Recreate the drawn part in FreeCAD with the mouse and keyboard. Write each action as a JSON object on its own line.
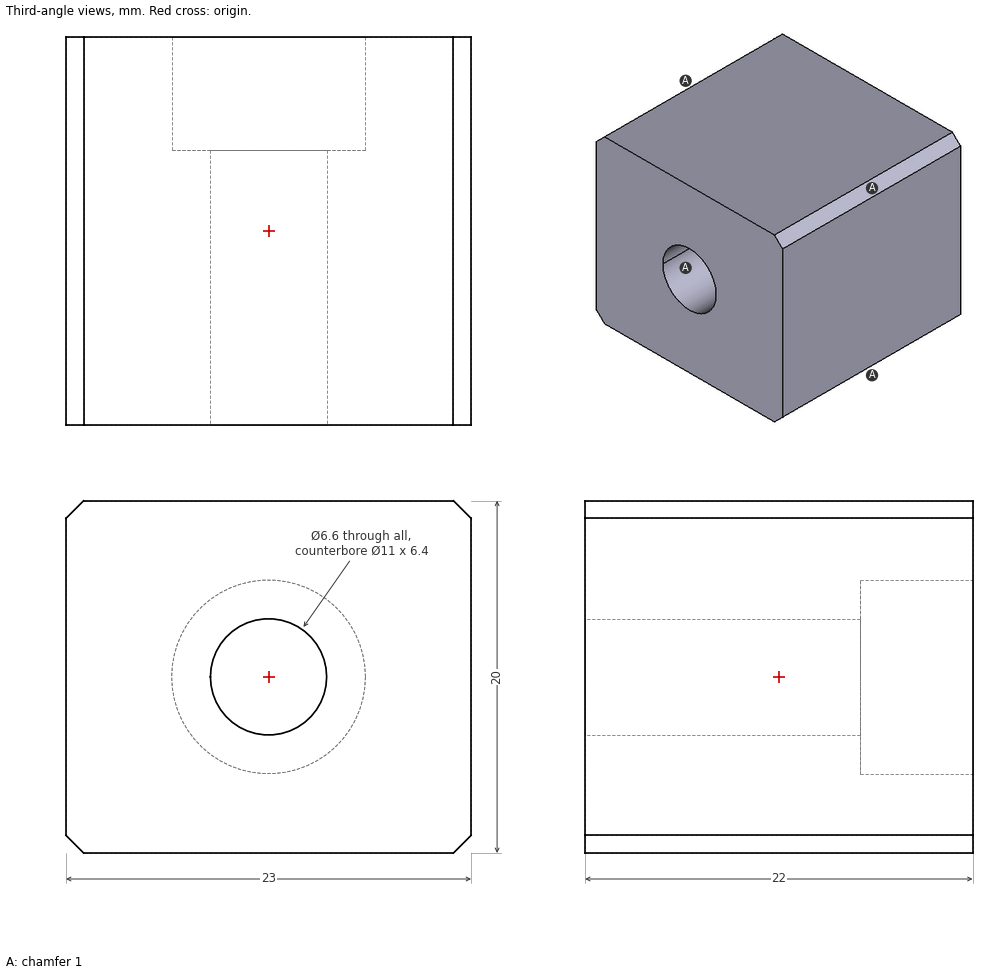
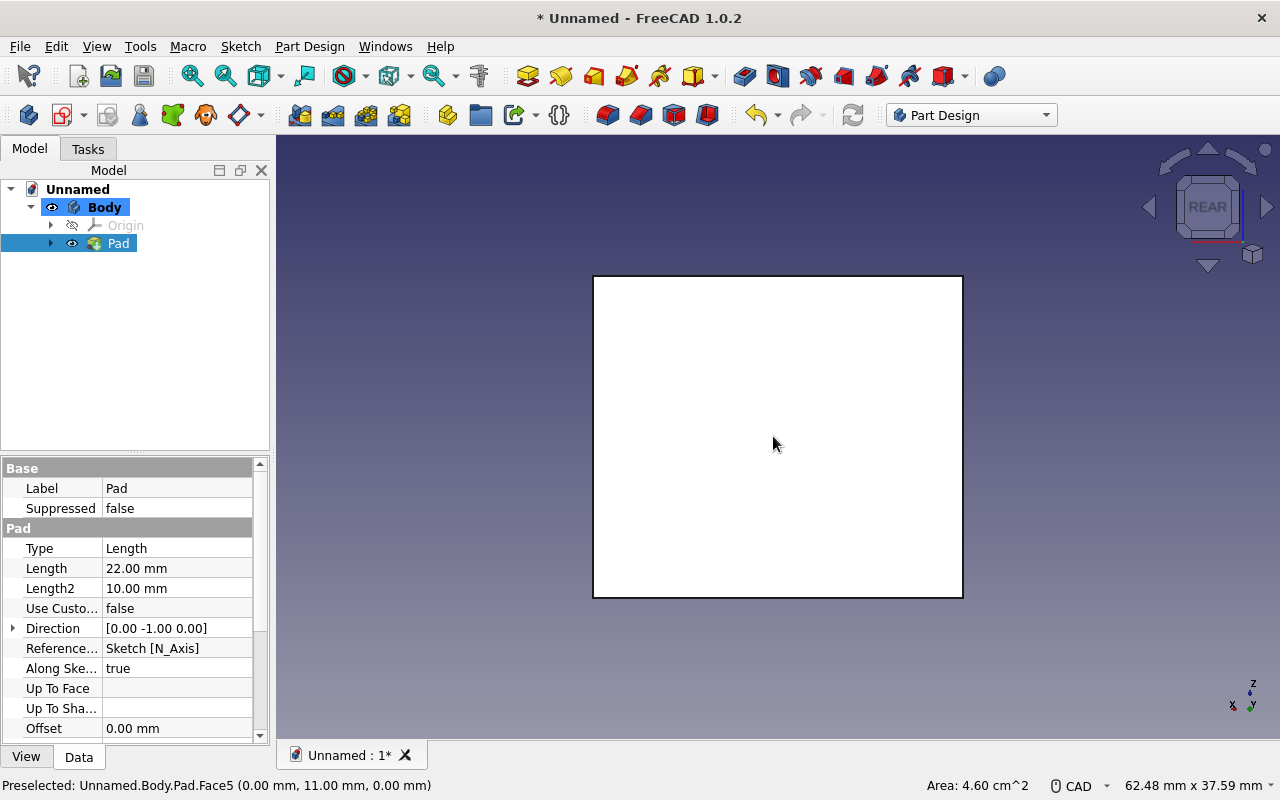
{"action": "left_click", "coordinate": [62, 116]}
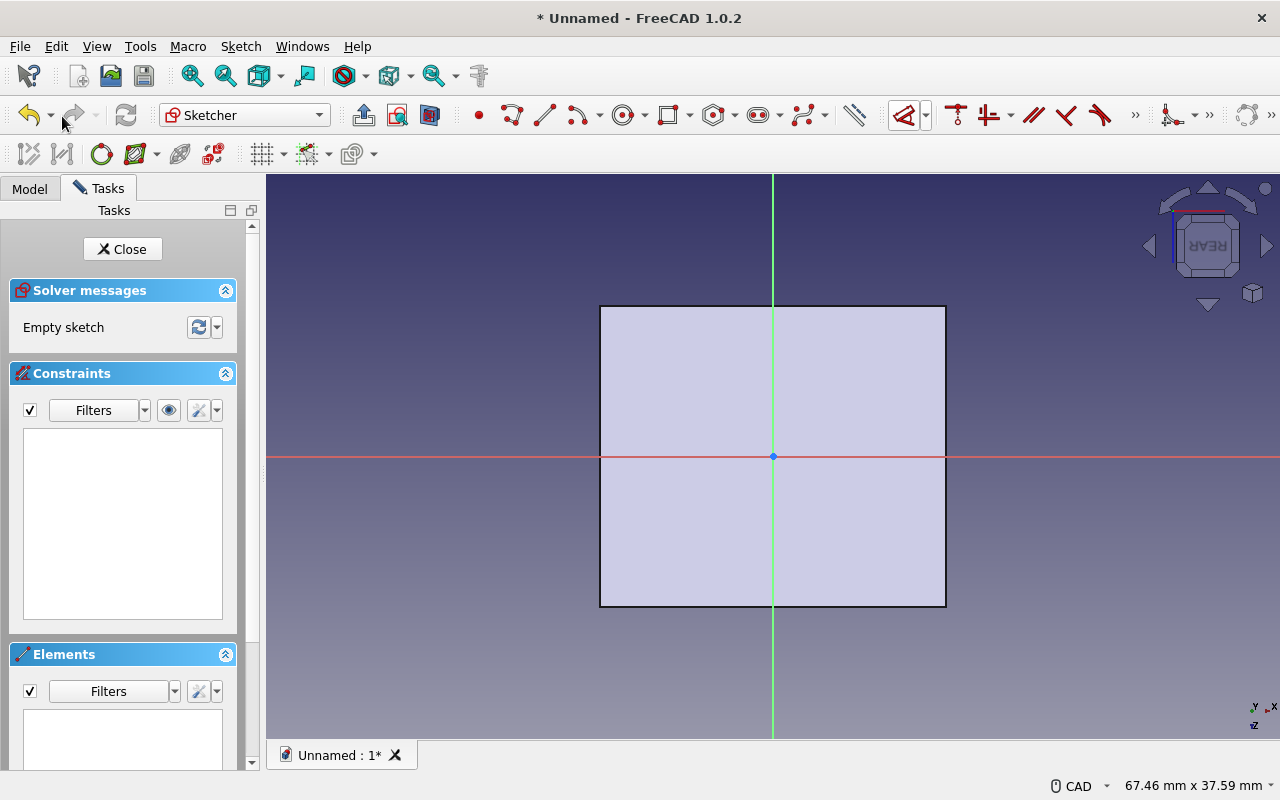
{"action": "scroll", "coordinate": [803, 457], "scroll_direction": "up", "scroll_amount": 6}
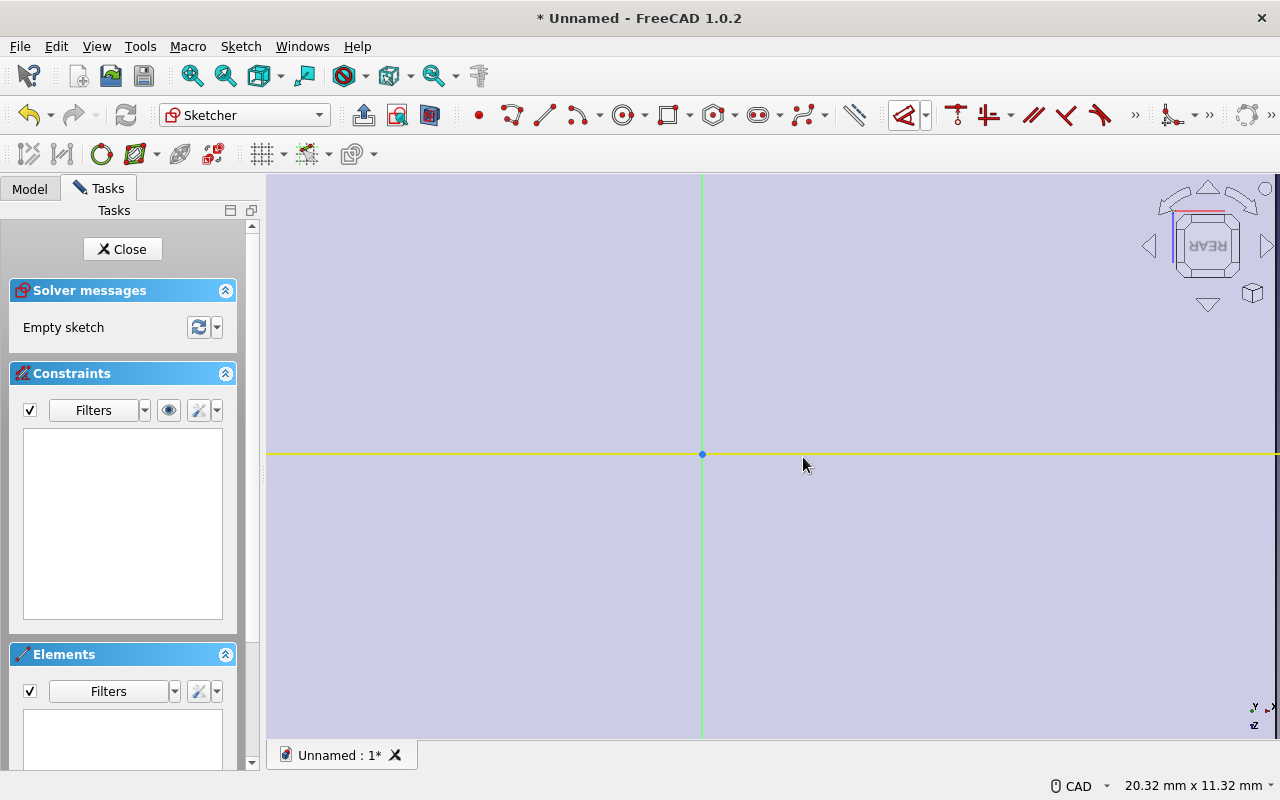
{"action": "left_click", "coordinate": [622, 116]}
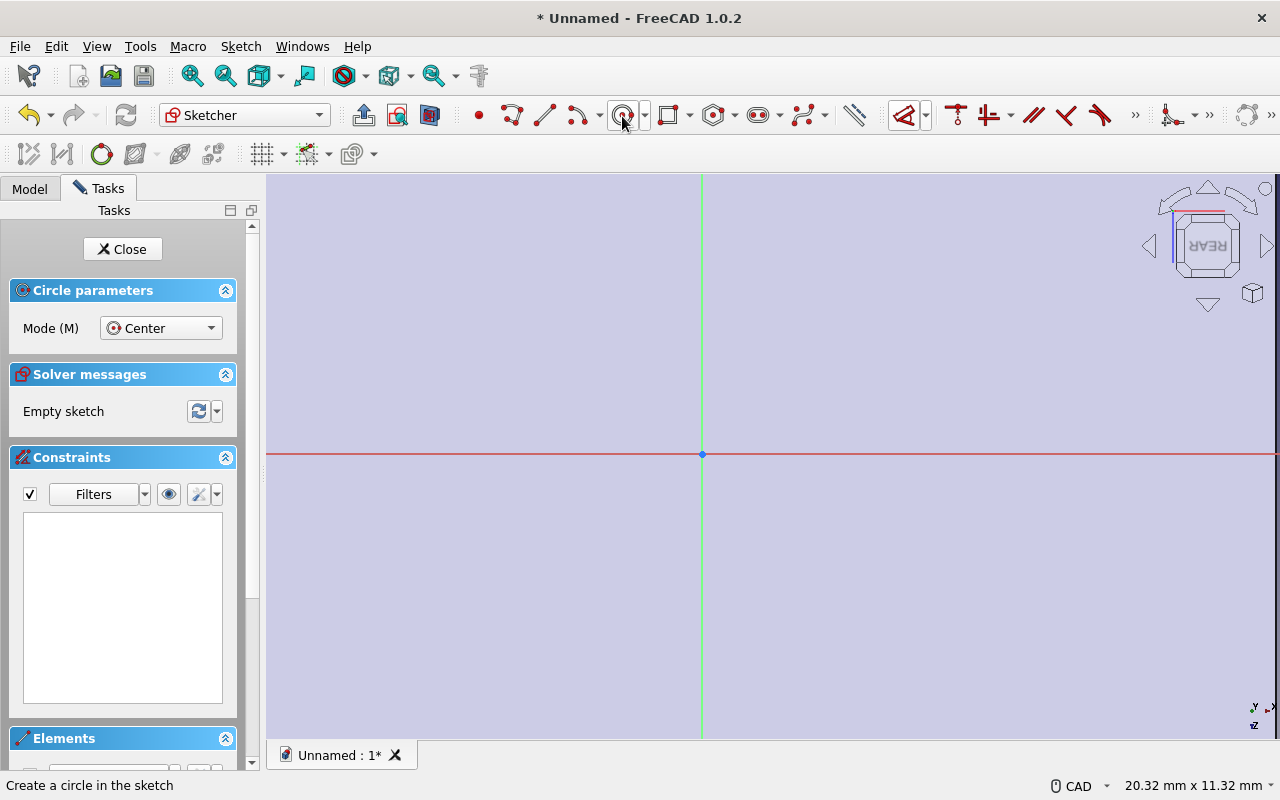
{"action": "left_click", "coordinate": [702, 454]}
{"action": "left_click", "coordinate": [819, 338]}
{"action": "key", "text": "Escape"}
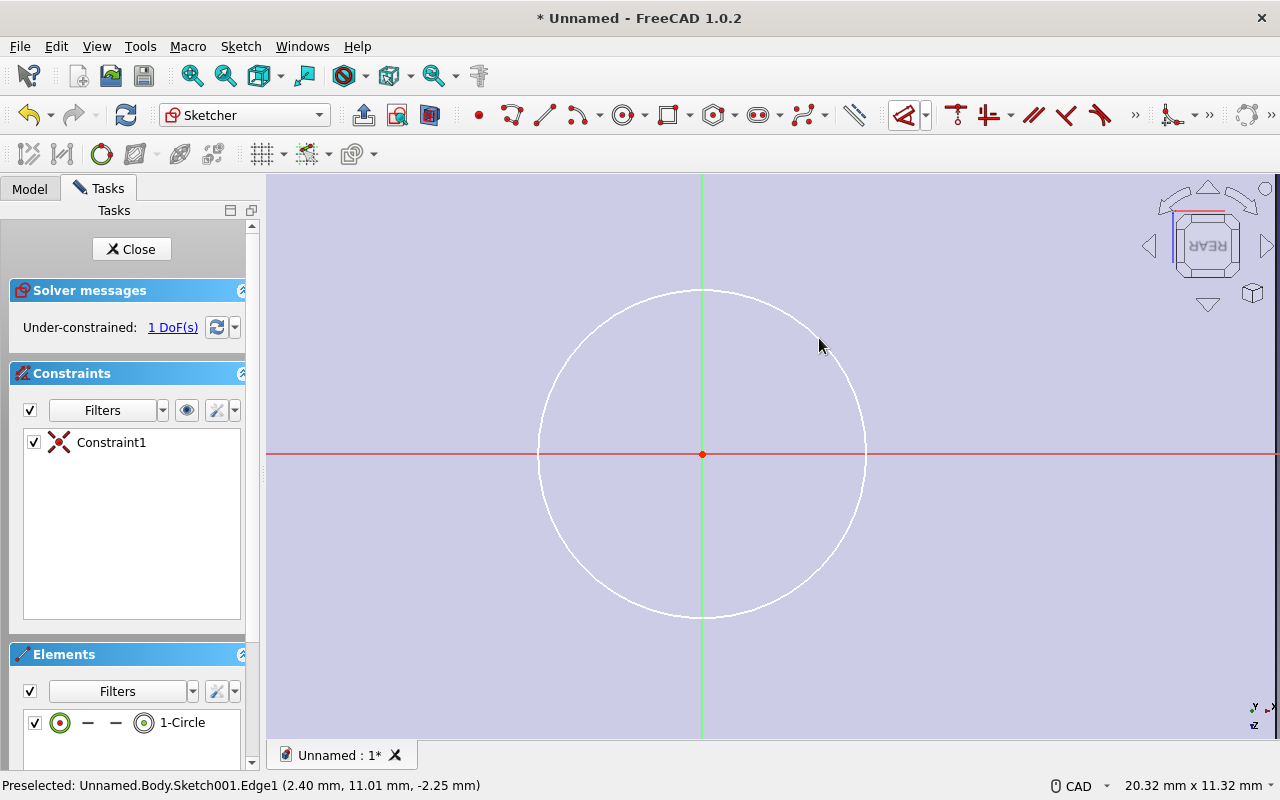
{"action": "left_click", "coordinate": [904, 116]}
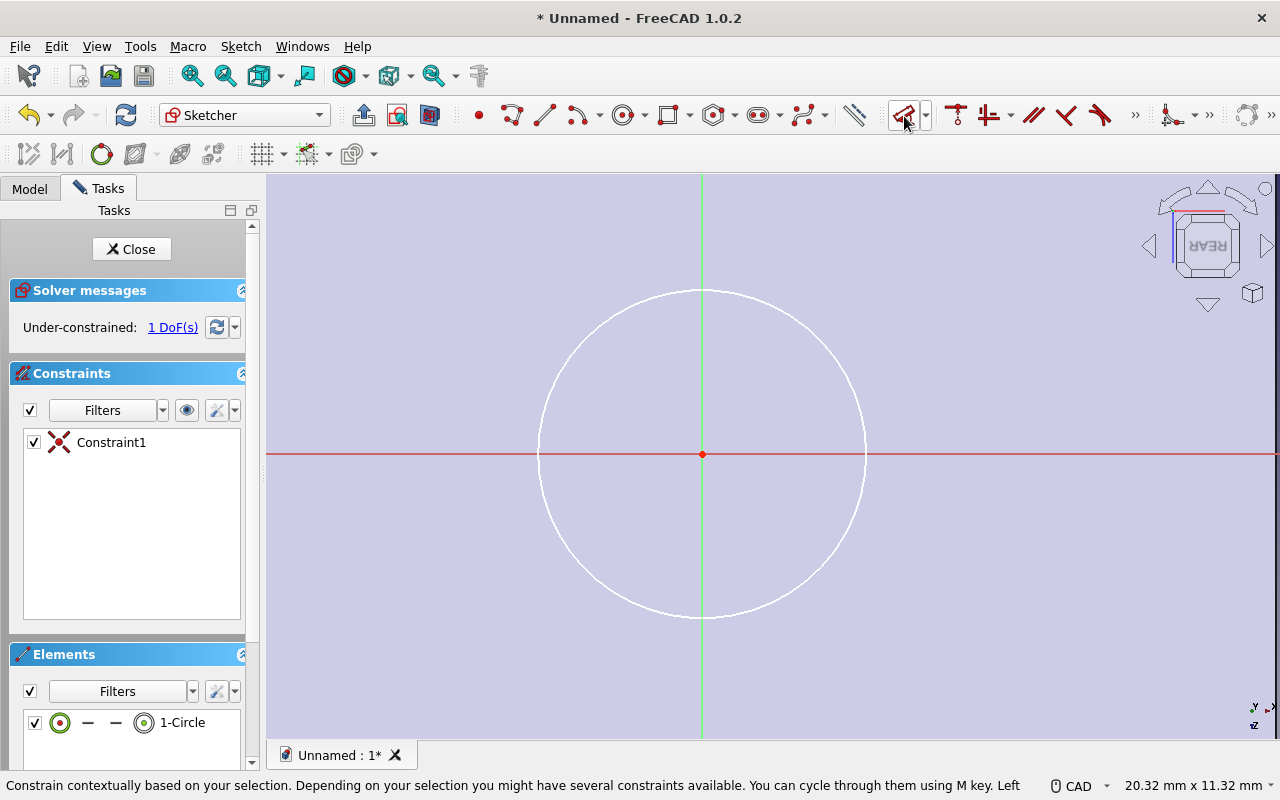
{"action": "left_click", "coordinate": [818, 338]}
{"action": "left_click", "coordinate": [841, 315]}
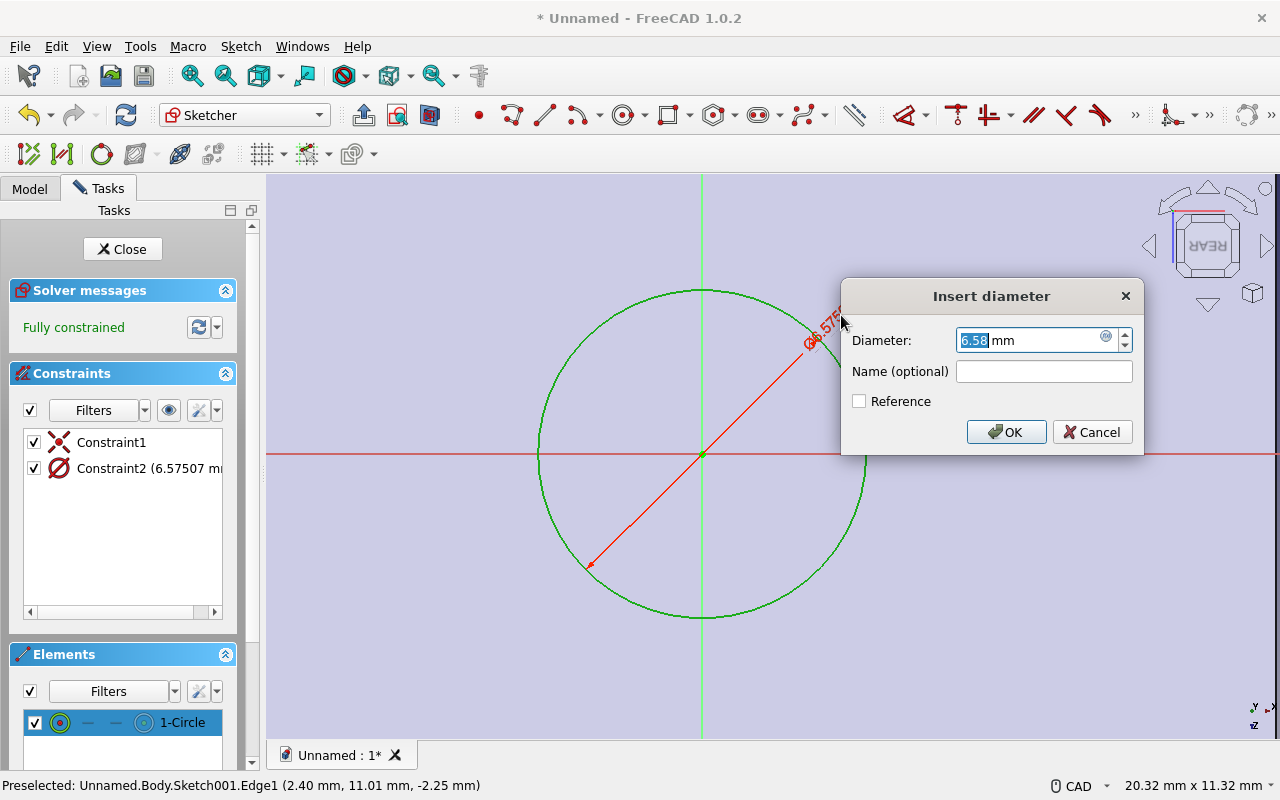
{"action": "type", "text": "6.6"}
{"action": "key", "text": "Return"}
{"action": "key", "text": "Escape"}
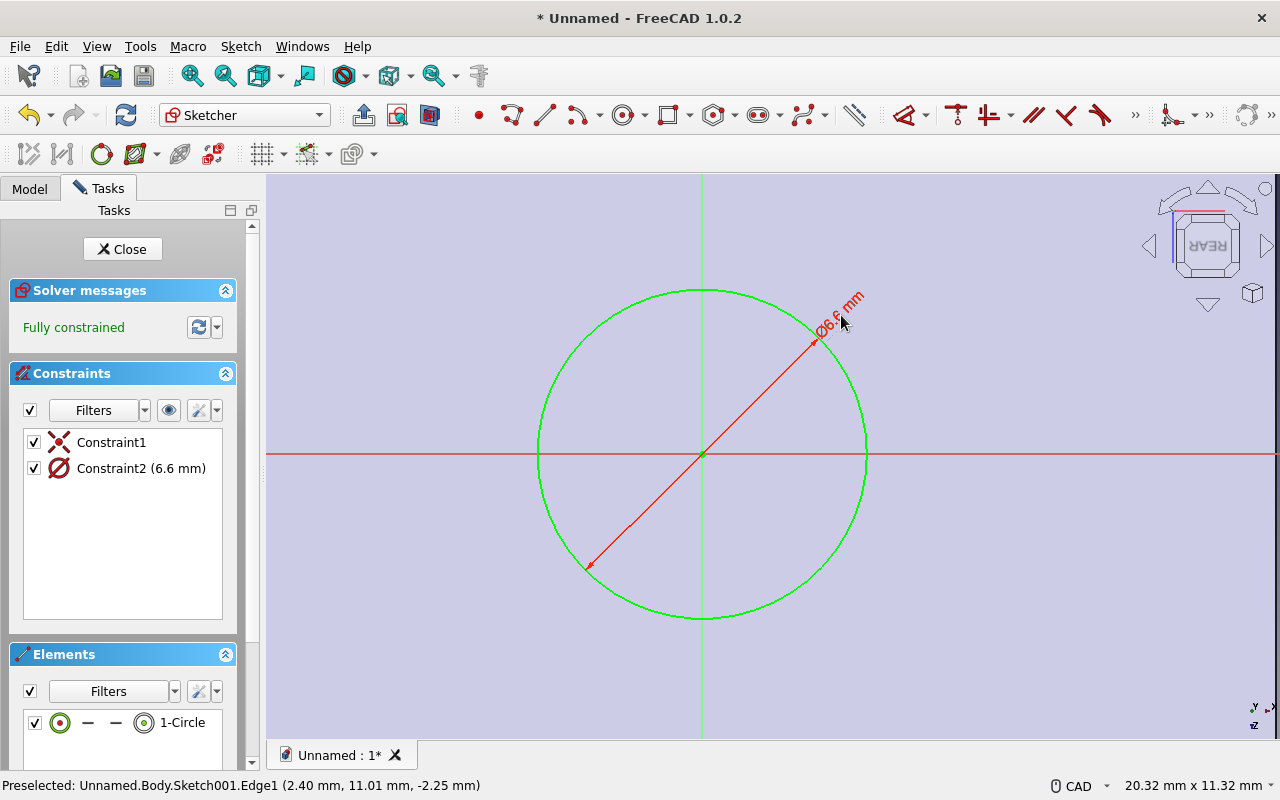
{"action": "left_click", "coordinate": [123, 249]}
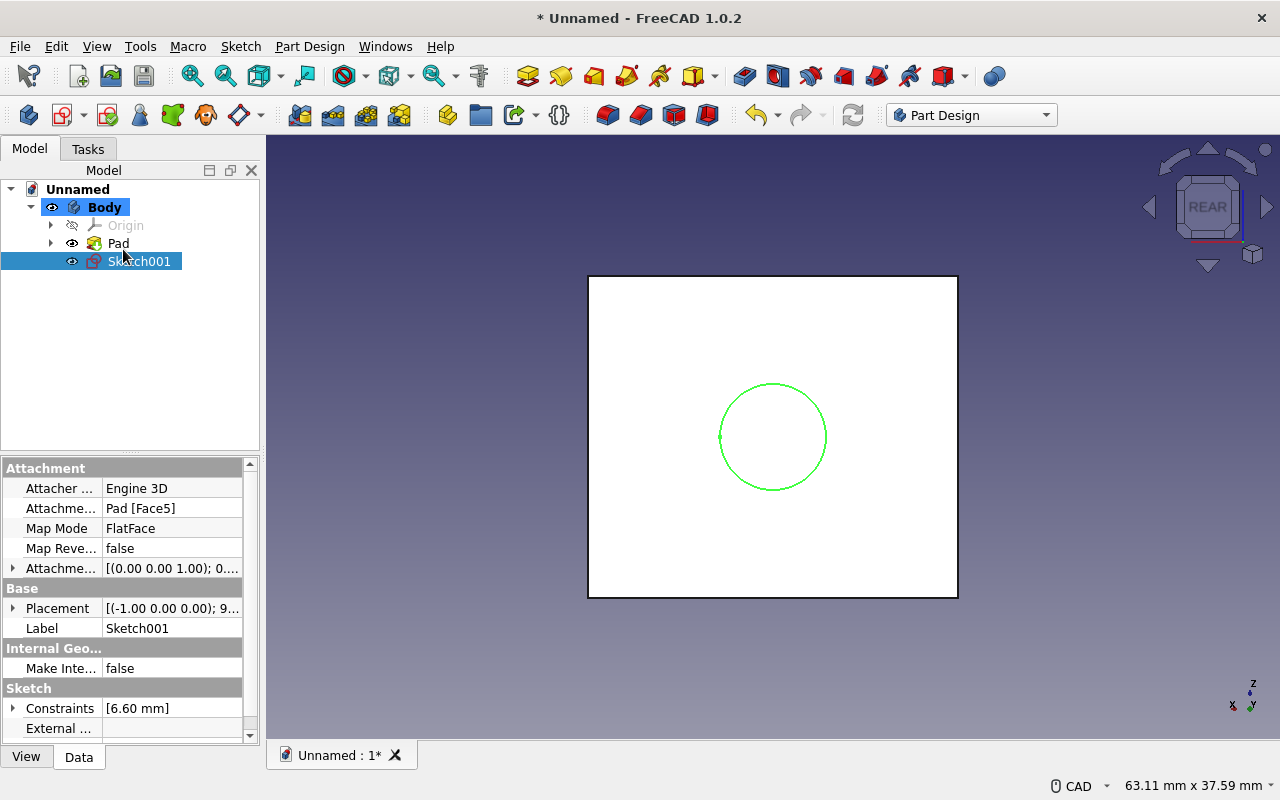
{"action": "left_click", "coordinate": [778, 76]}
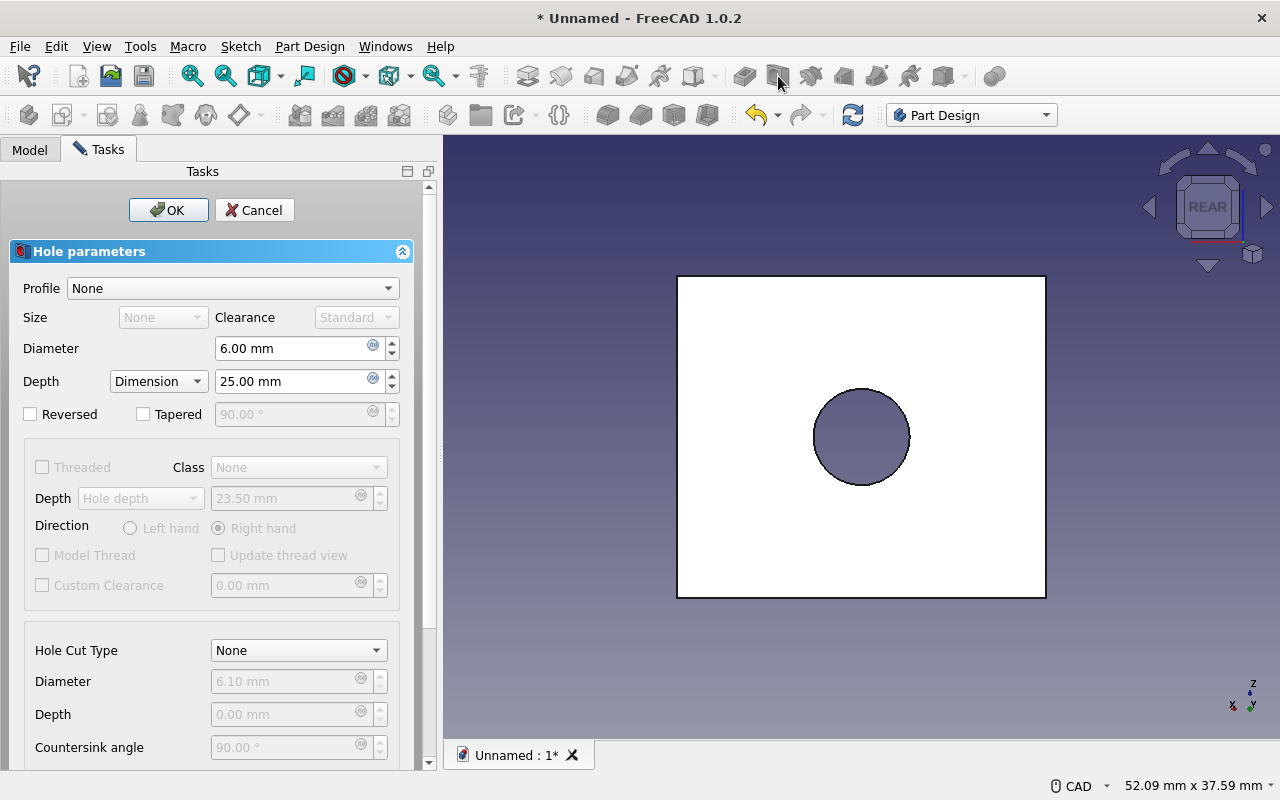
{"action": "triple_click", "coordinate": [300, 348]}